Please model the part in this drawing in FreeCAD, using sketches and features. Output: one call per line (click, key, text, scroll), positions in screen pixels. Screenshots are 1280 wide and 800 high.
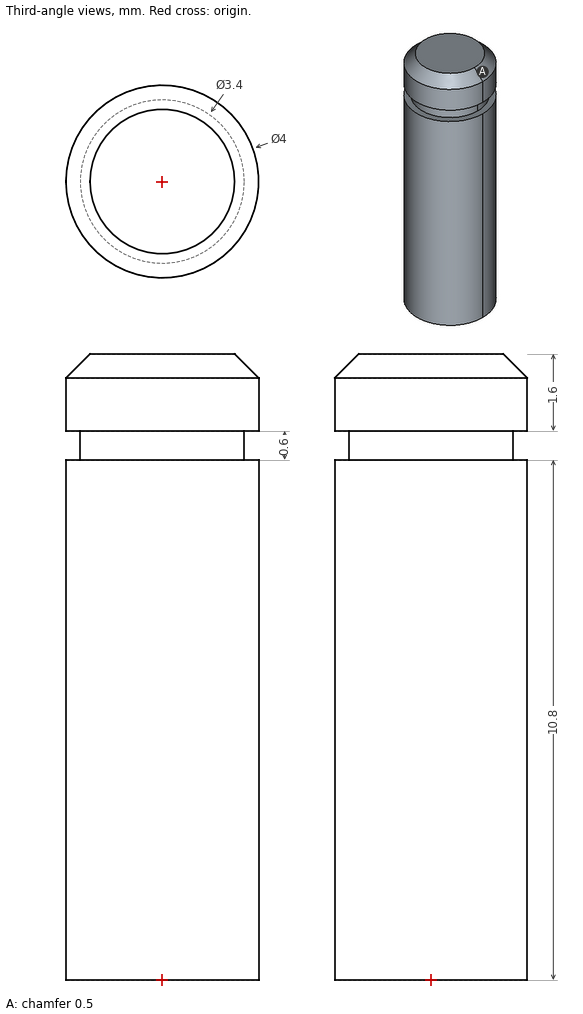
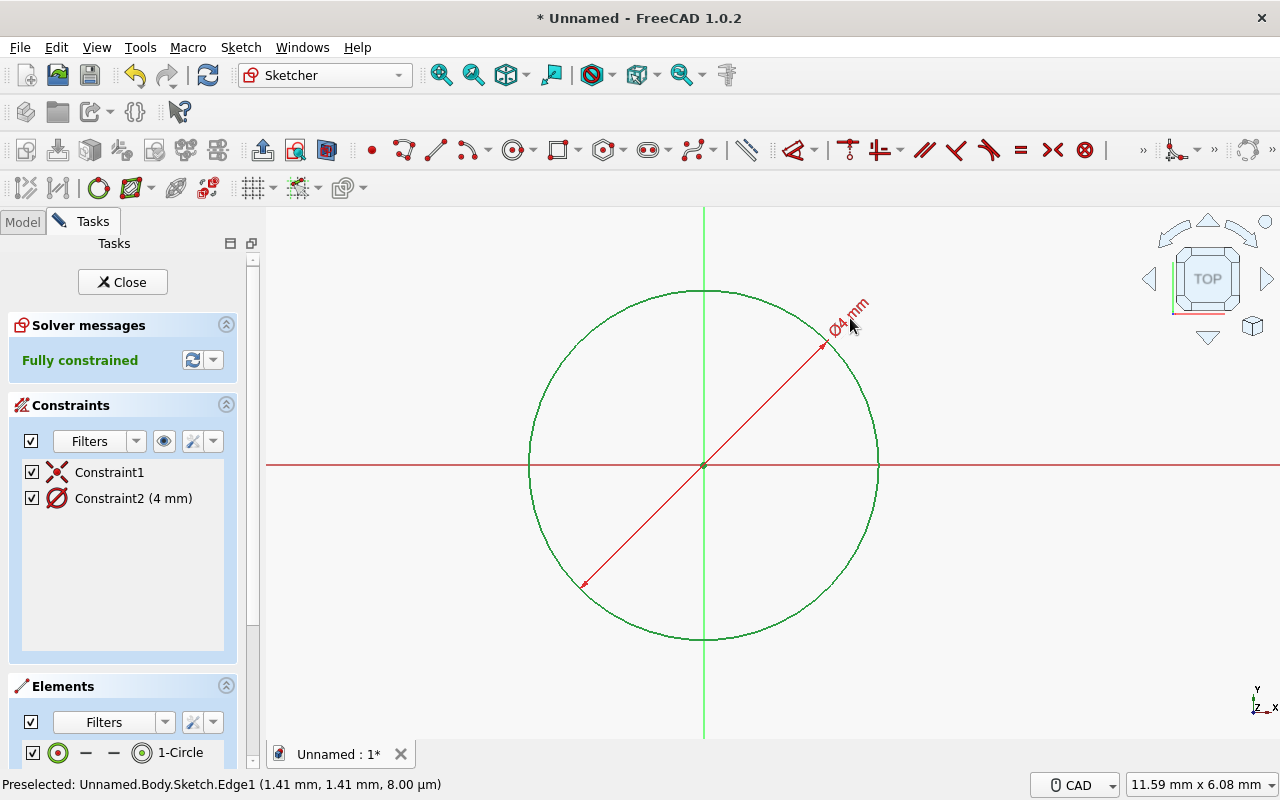
click(123, 282)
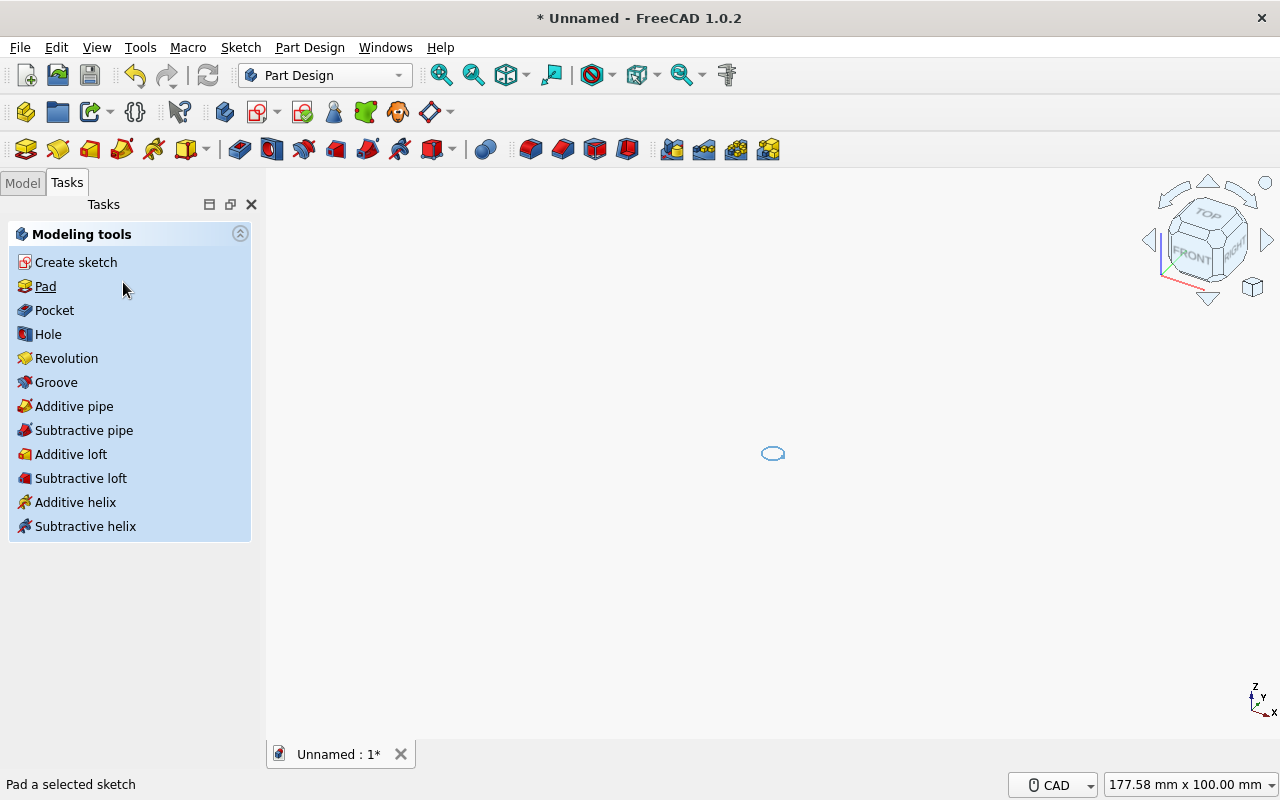
click(26, 150)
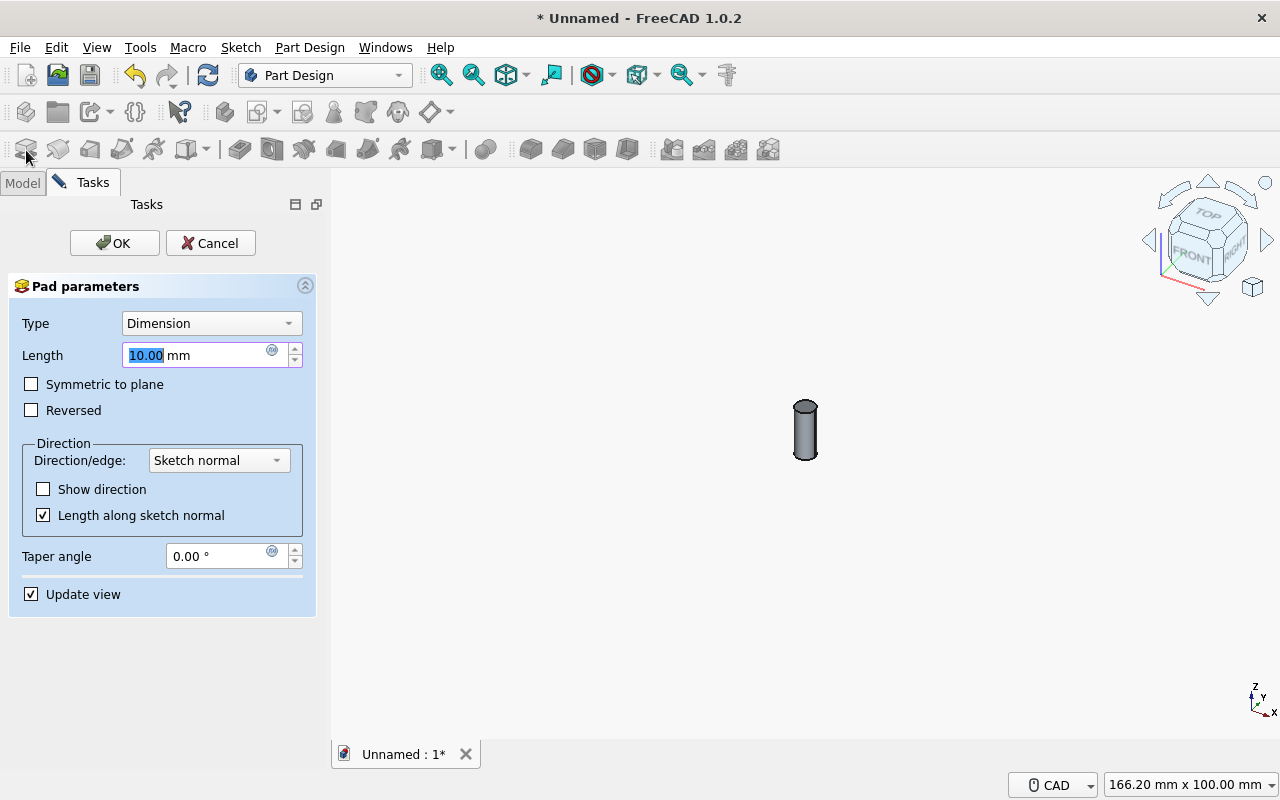
text(10.8)
key(Tab)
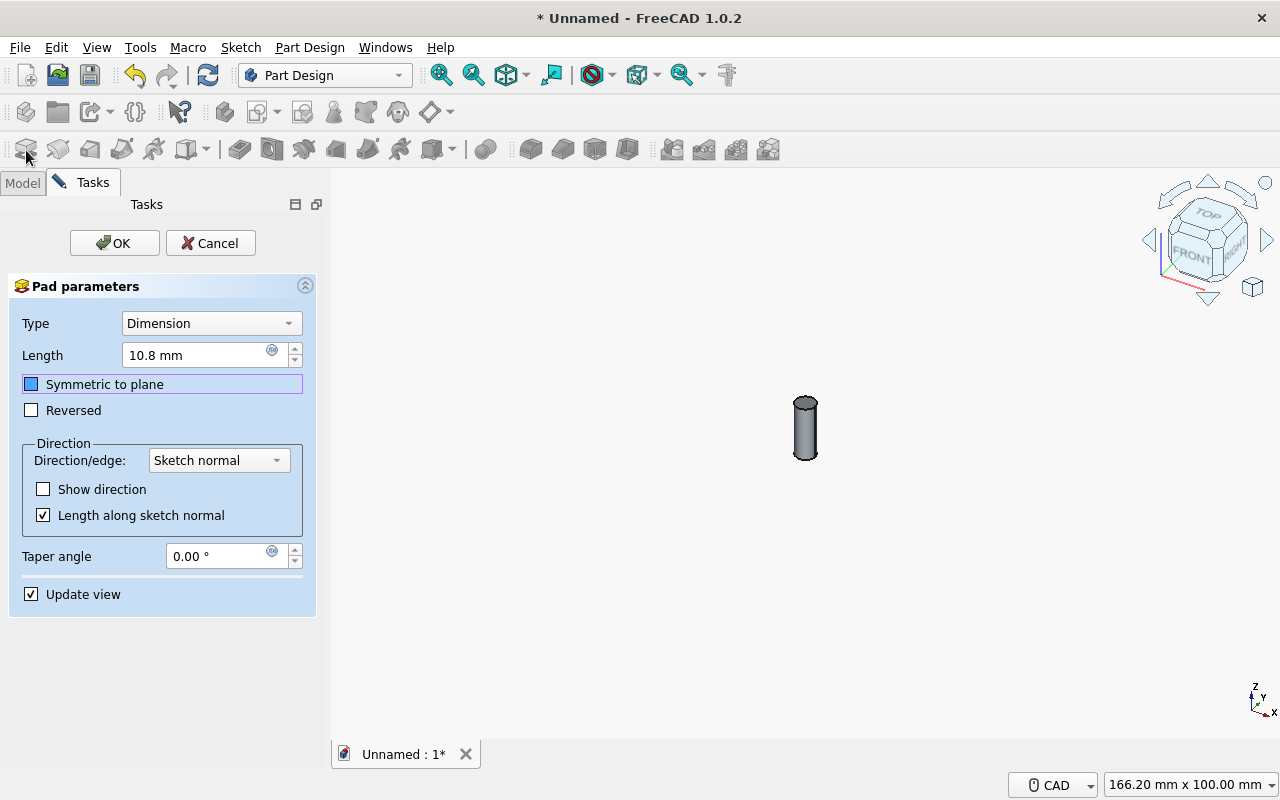
click(115, 243)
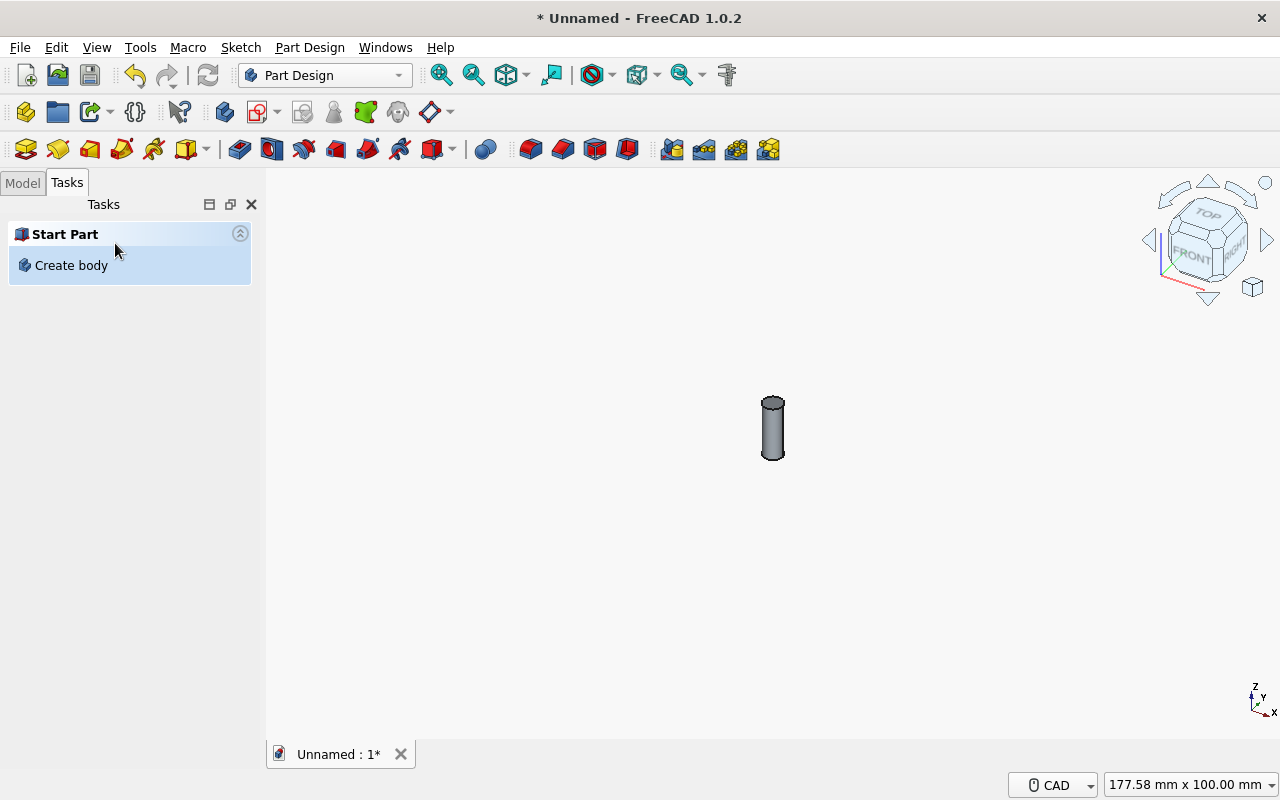
key(v)
key(f)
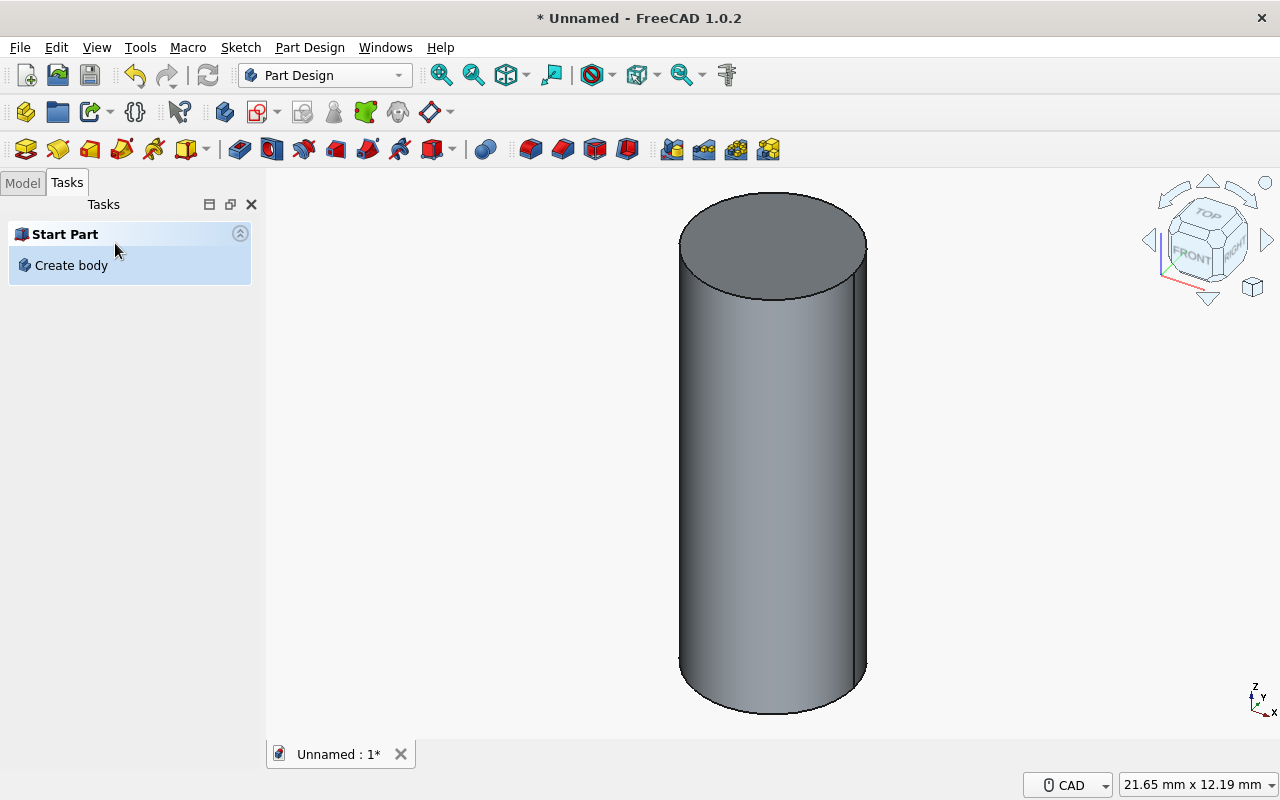
click(773, 245)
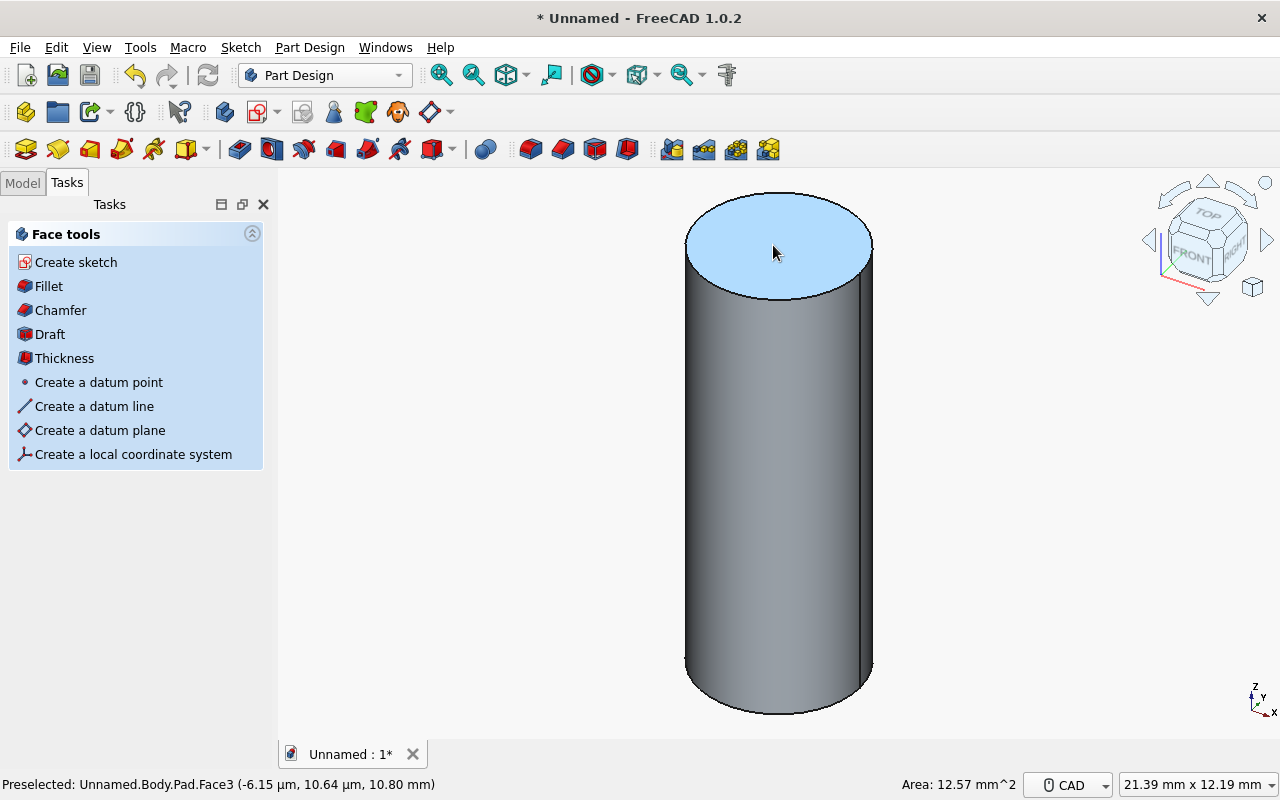
click(258, 112)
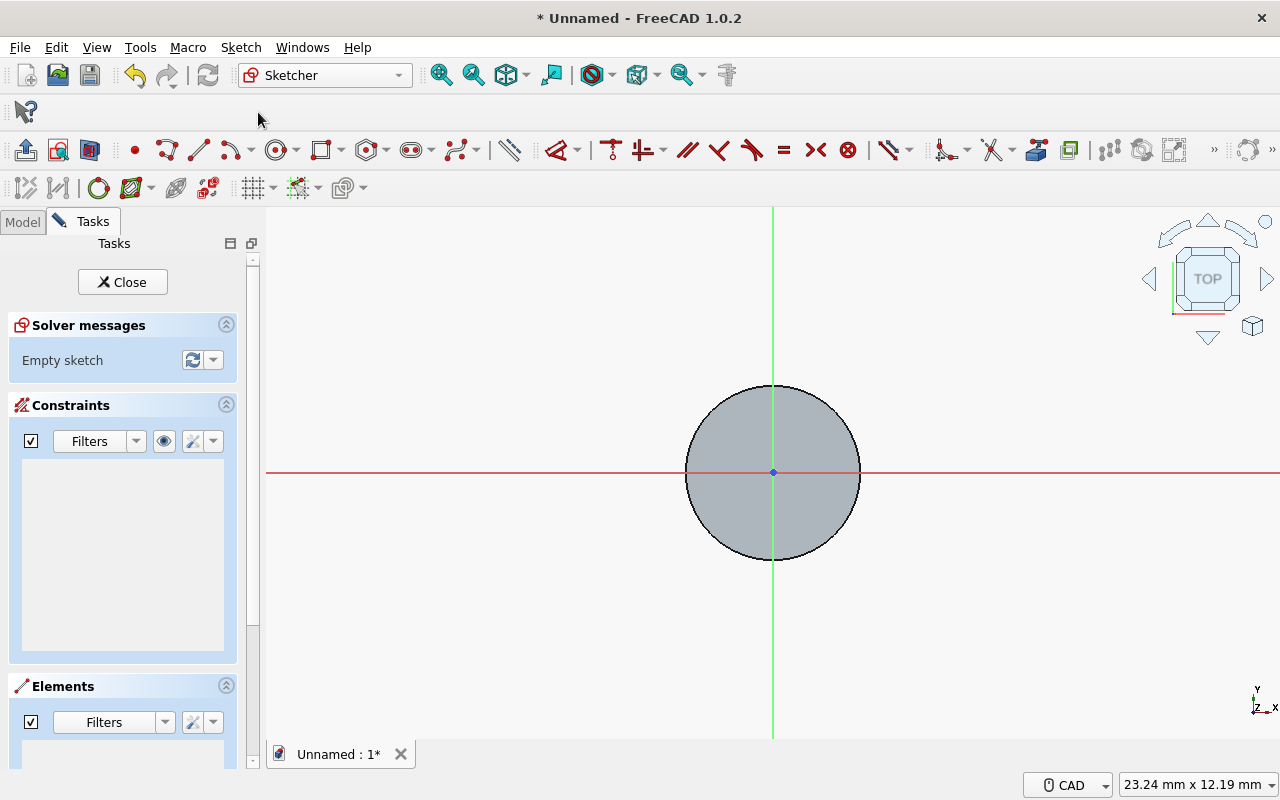
scroll(829, 473, up, 4)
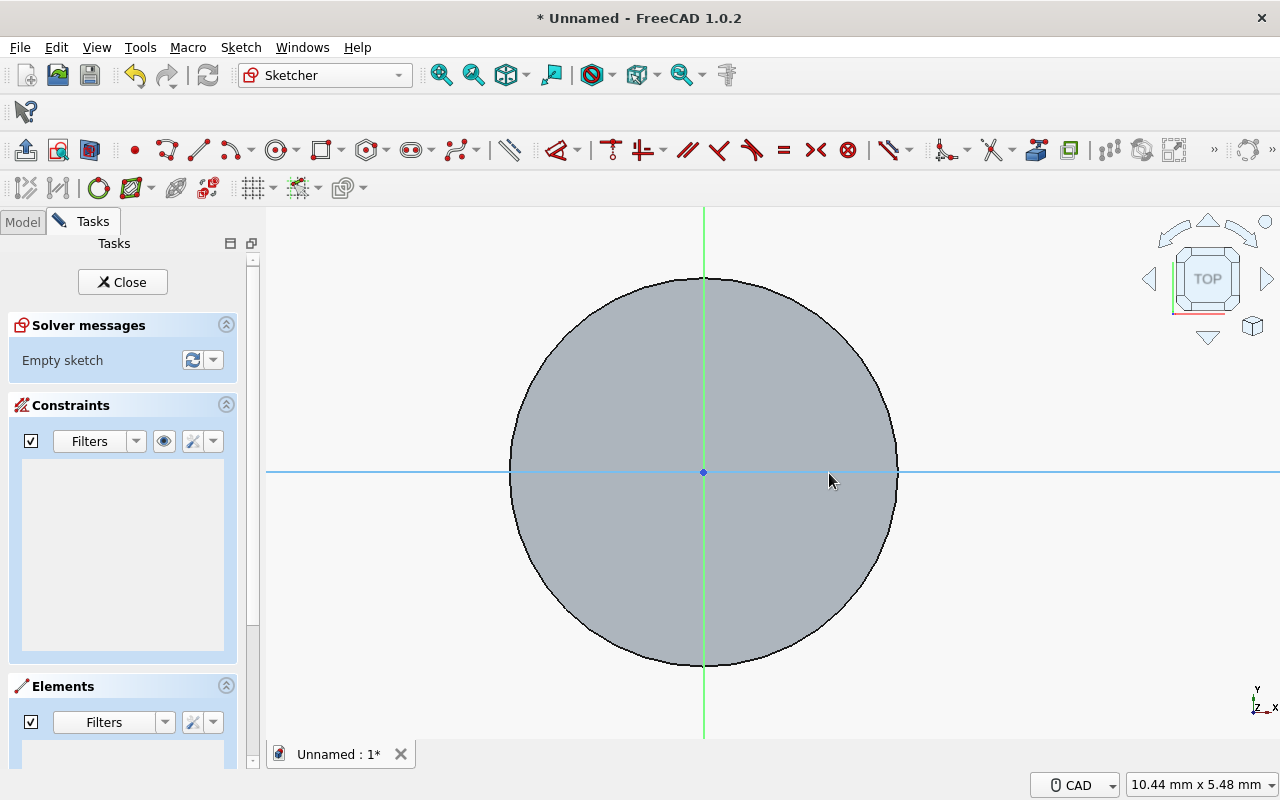
key(g)
key(c)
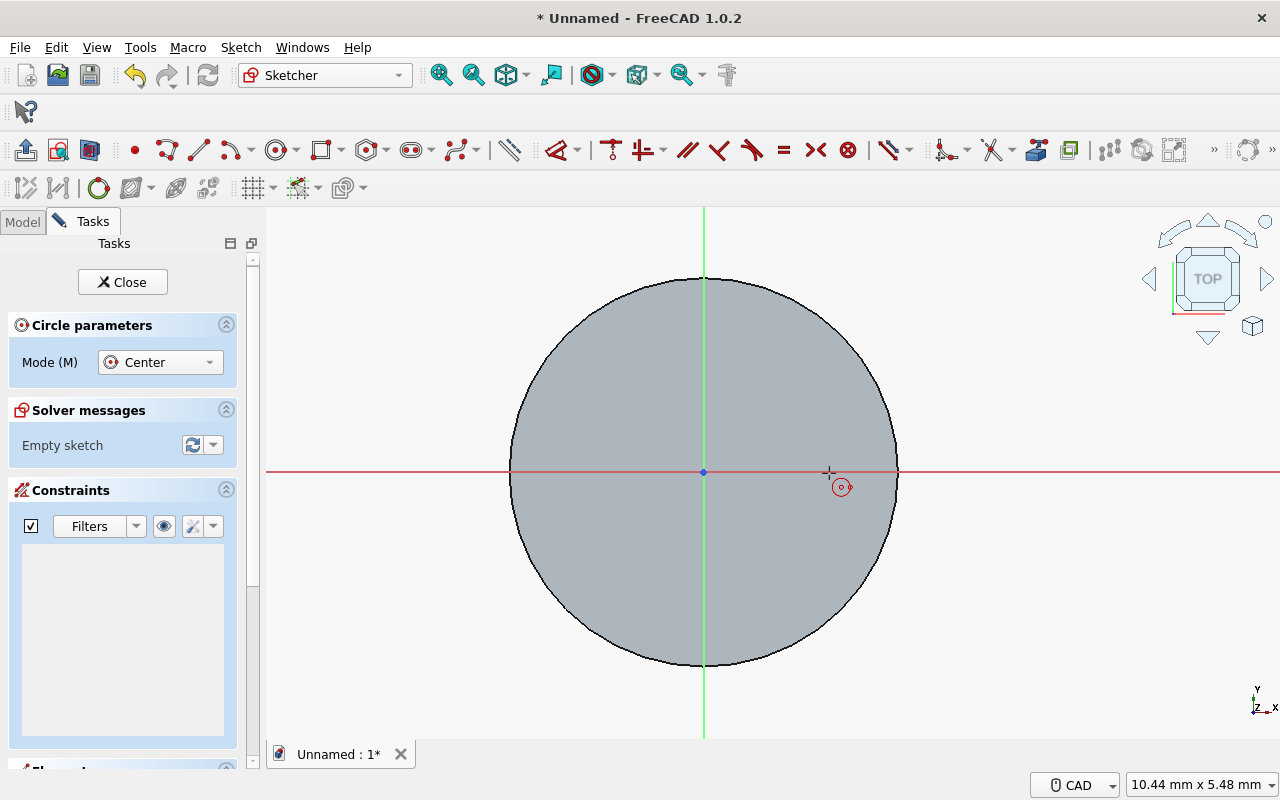
click(704, 472)
click(820, 356)
key(Escape)